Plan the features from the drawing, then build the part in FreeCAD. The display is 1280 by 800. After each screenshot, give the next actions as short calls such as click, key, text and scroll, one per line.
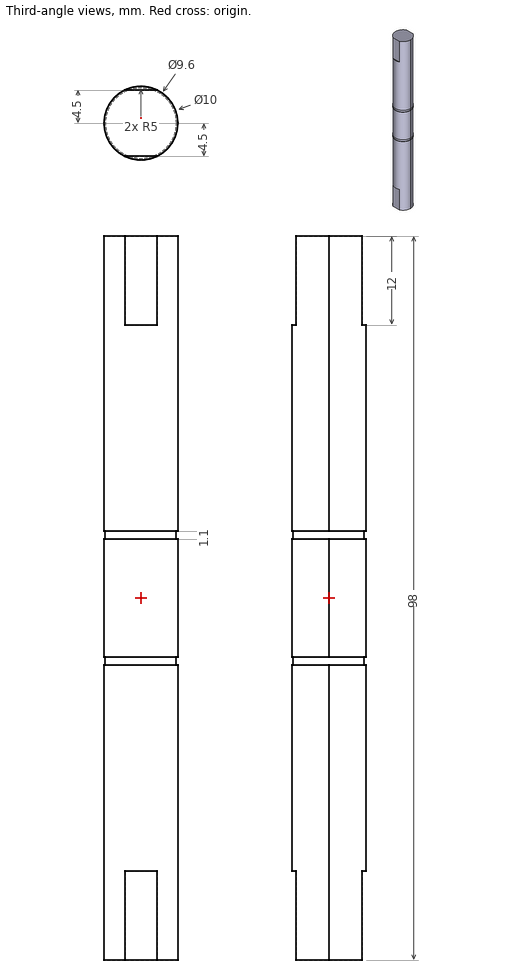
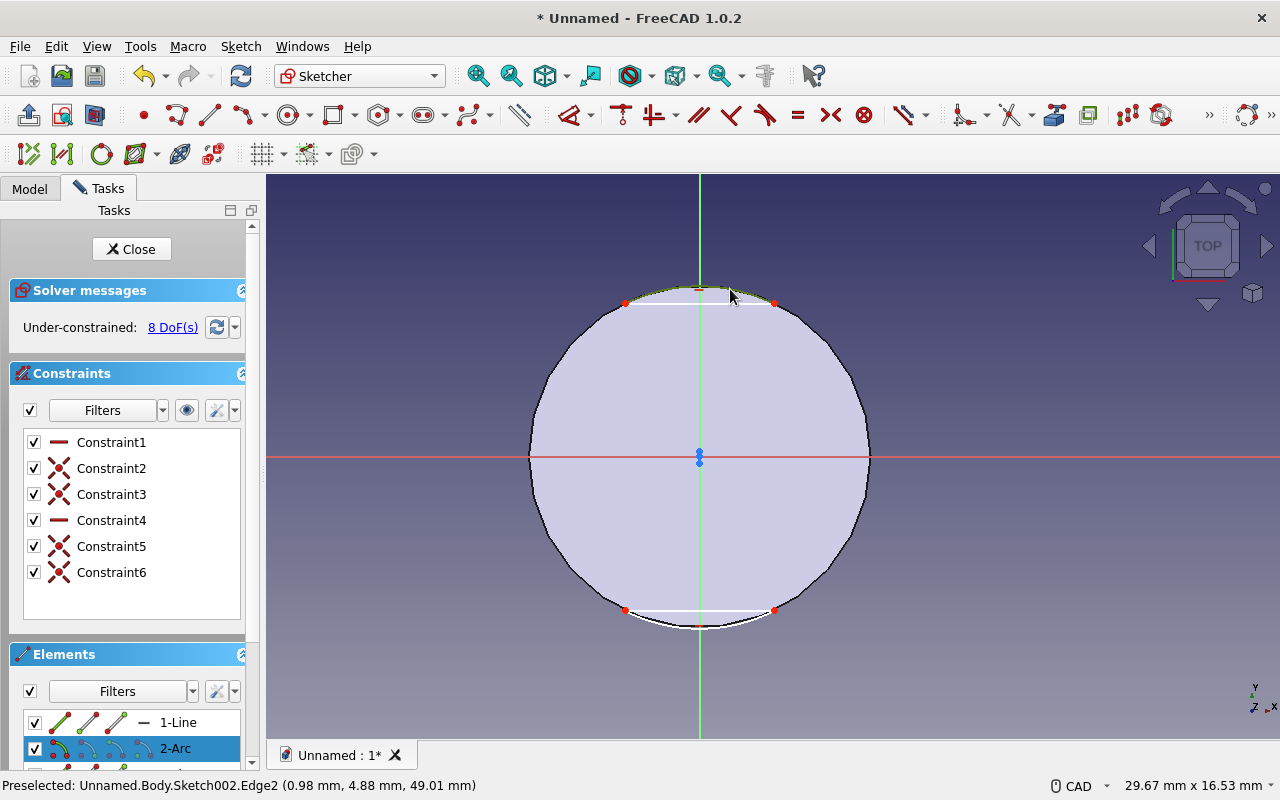
click(669, 626)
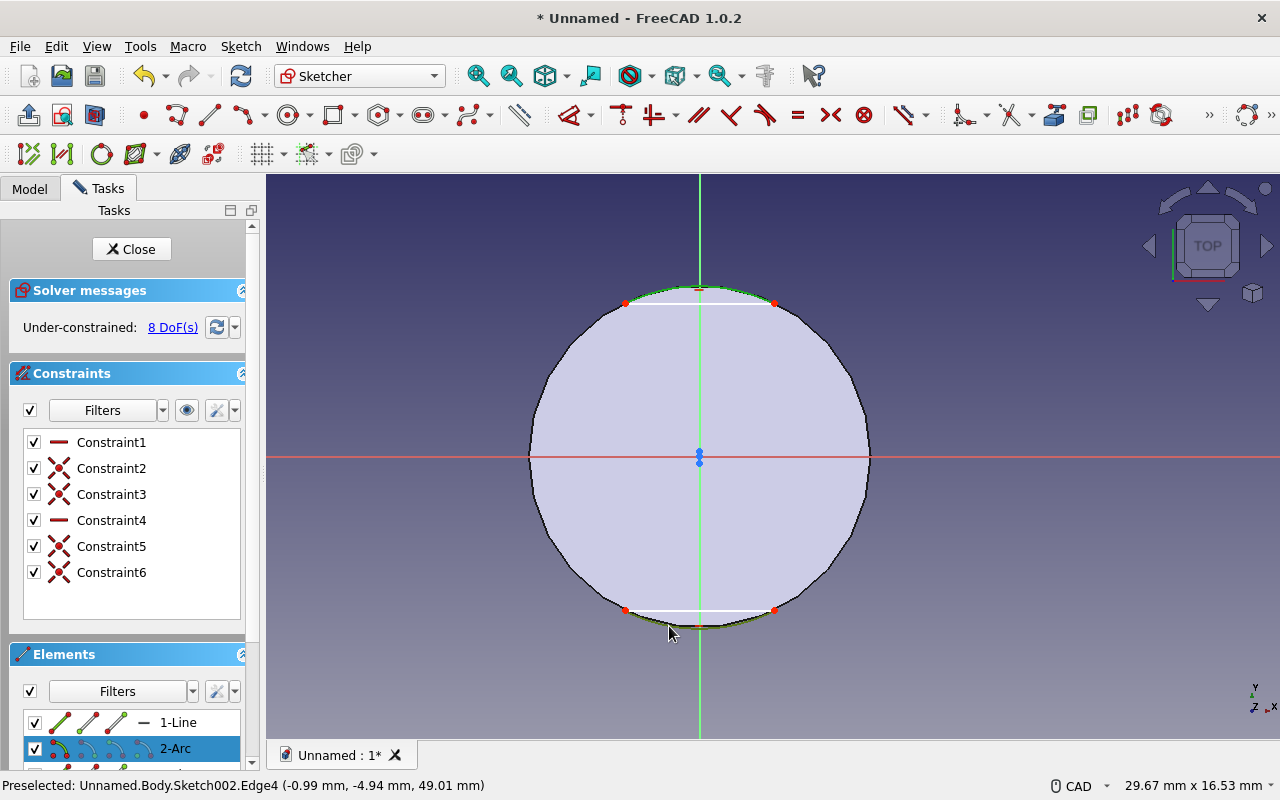
click(621, 116)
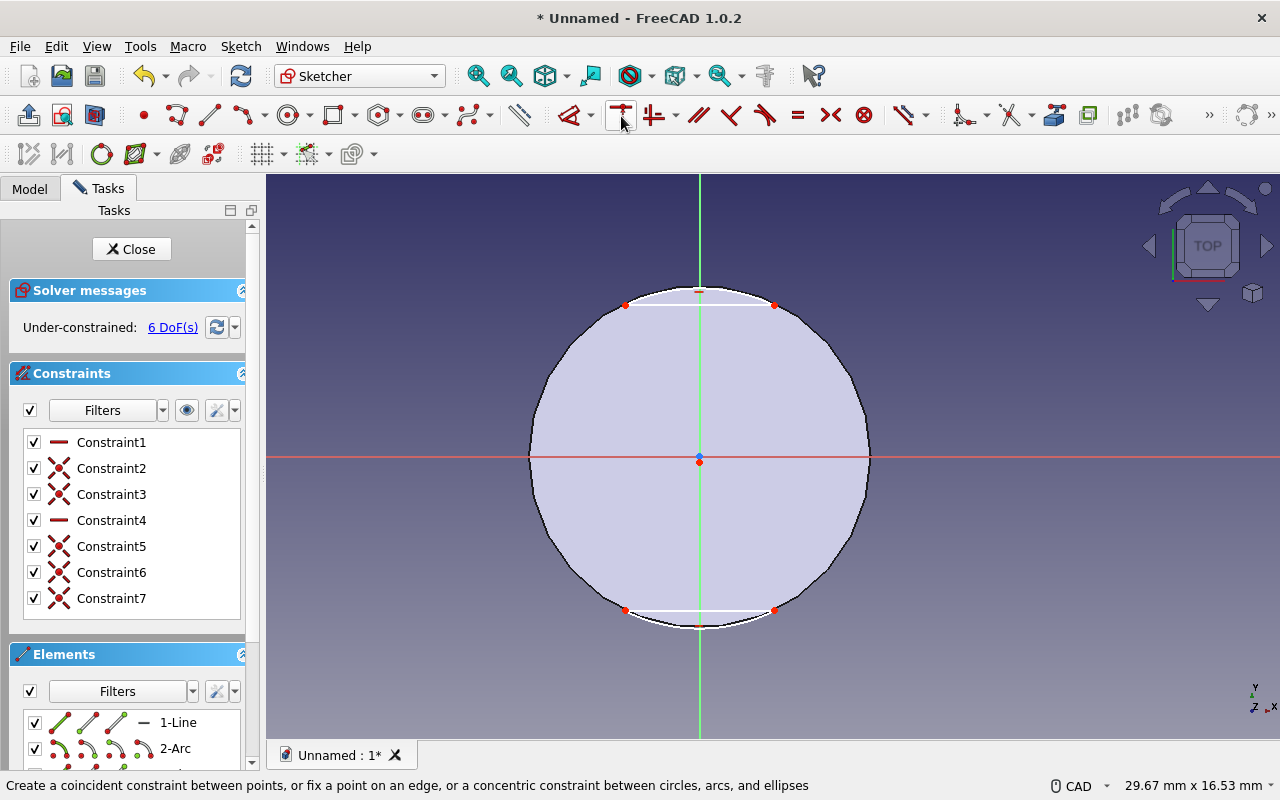
drag(690, 446, 710, 472)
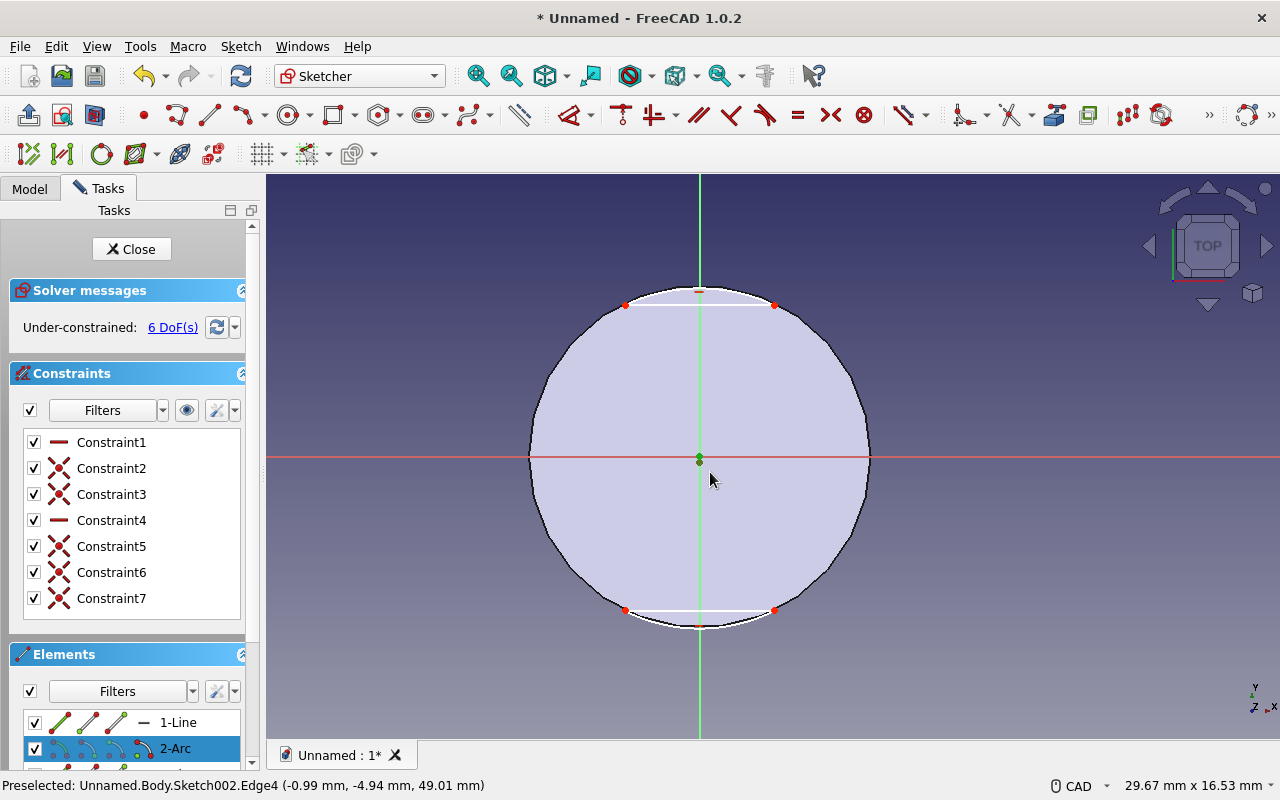
click(621, 116)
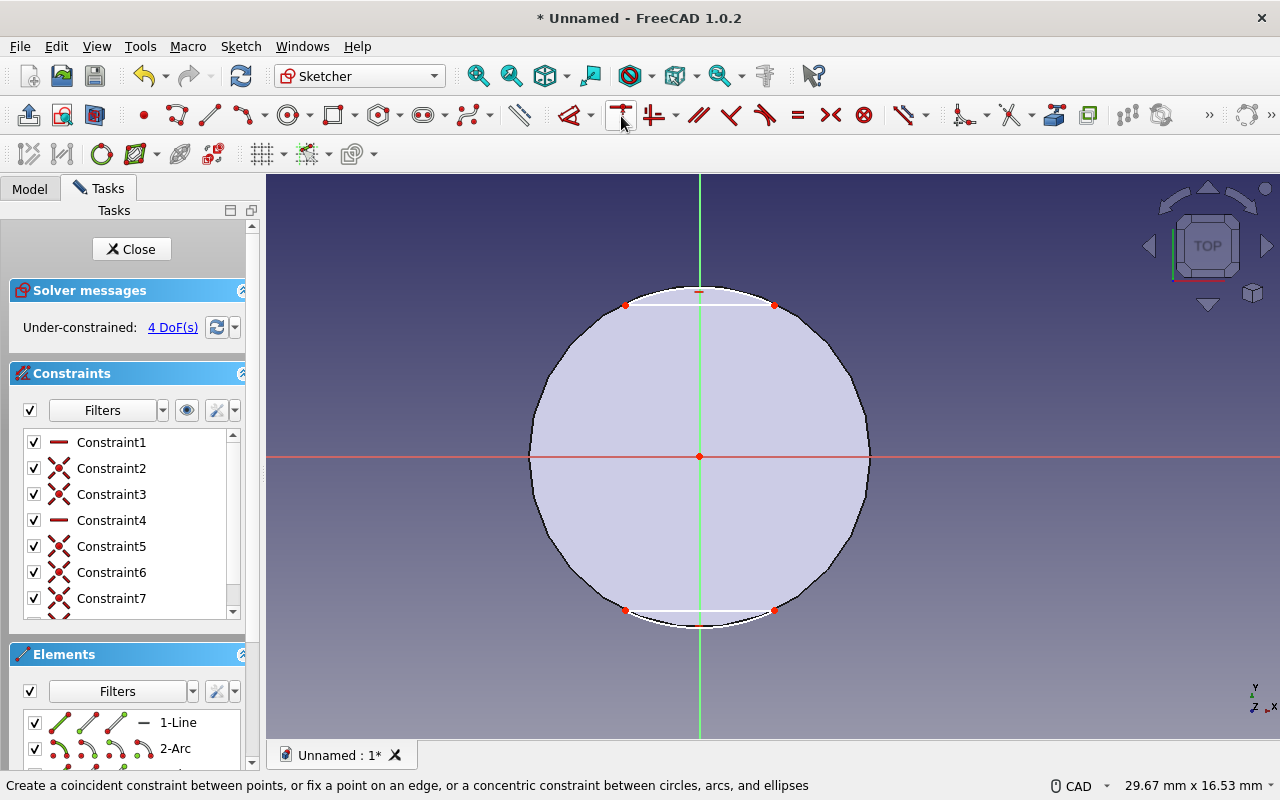
click(730, 291)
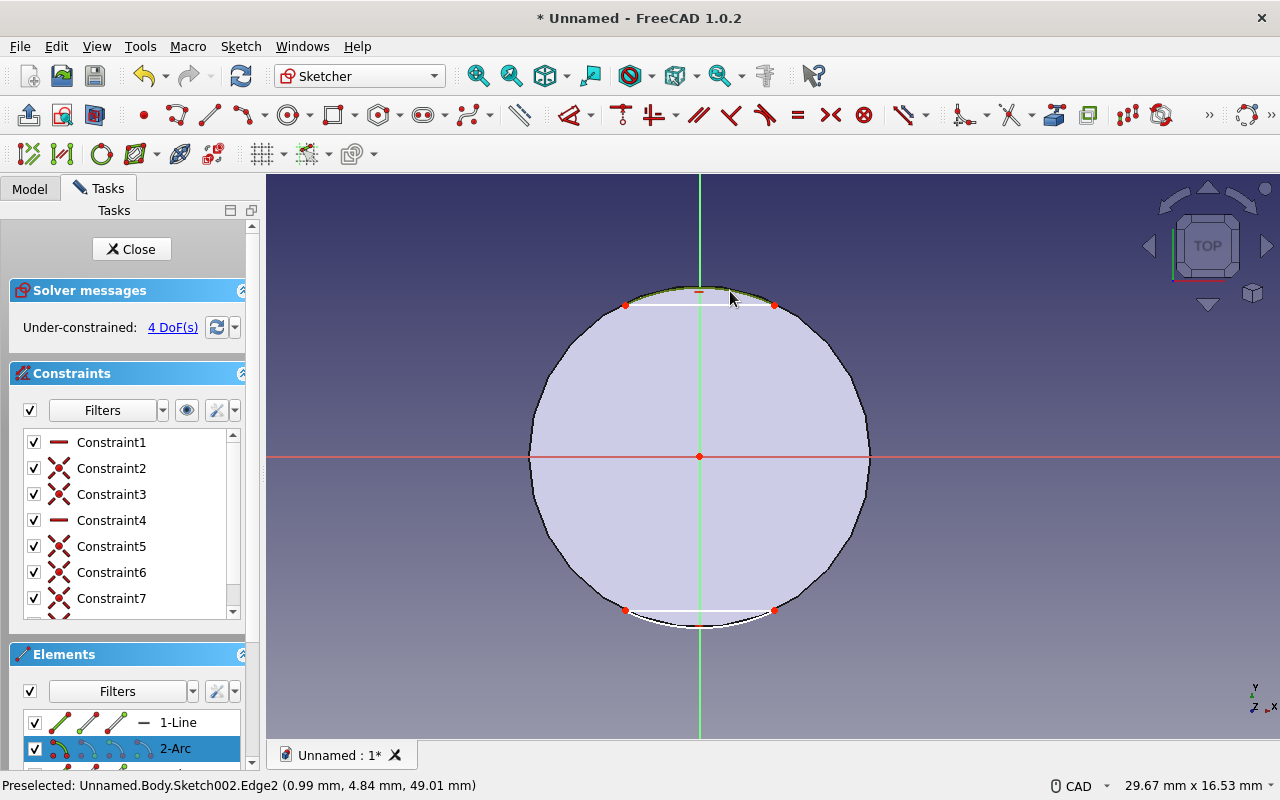
click(669, 625)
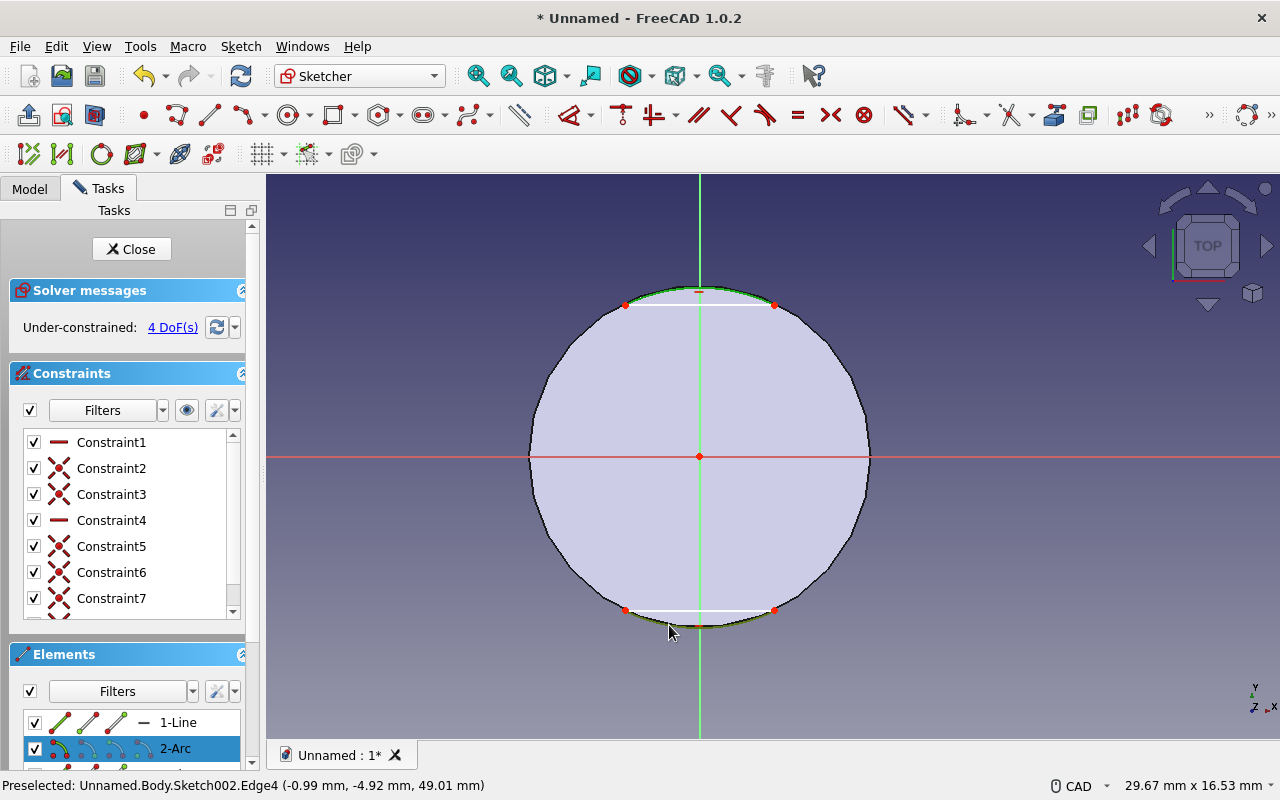
click(798, 116)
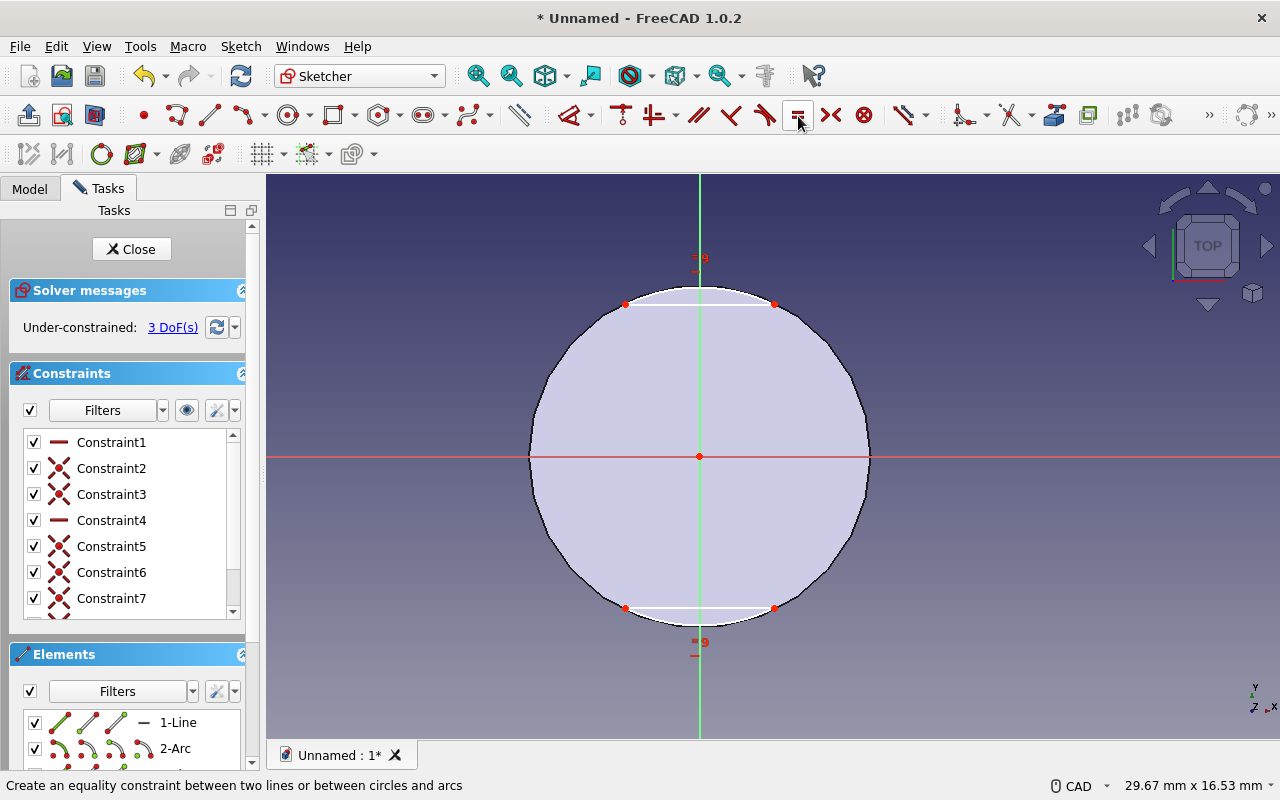
click(568, 116)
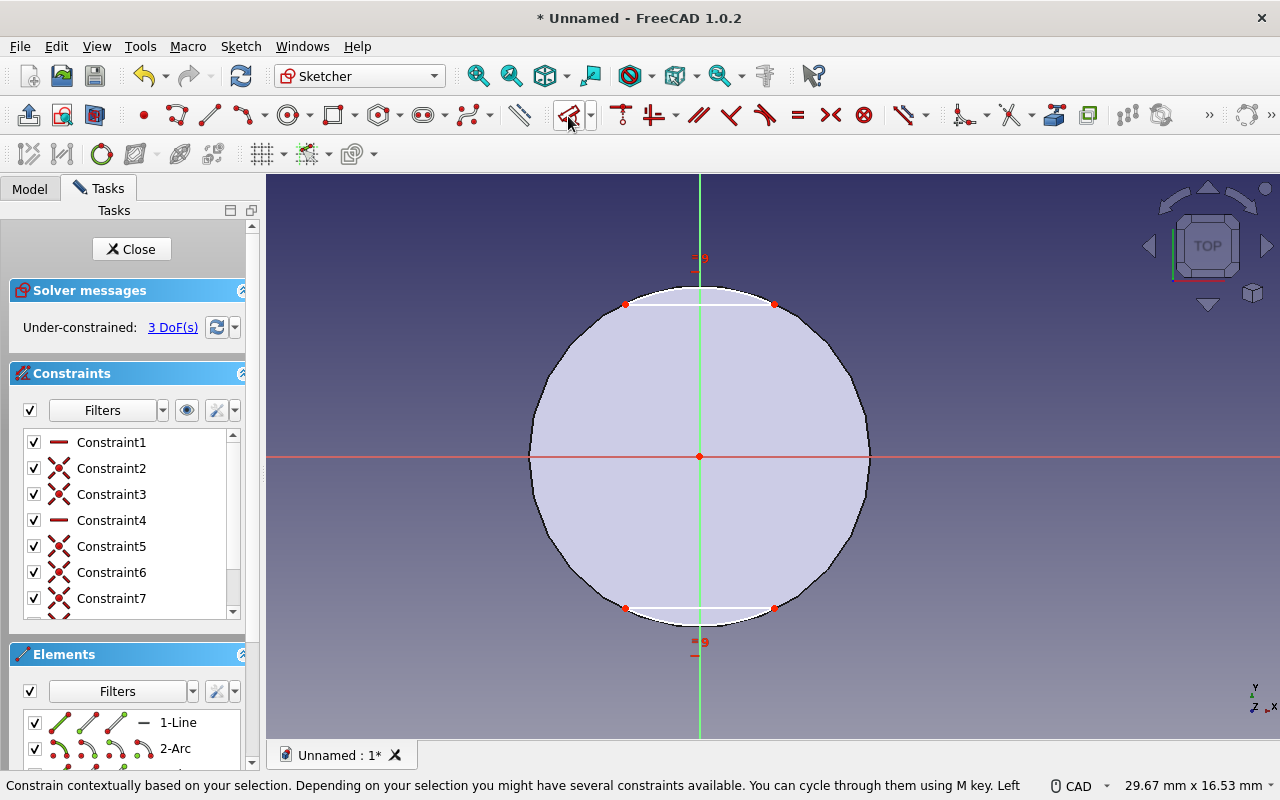
click(730, 290)
click(736, 259)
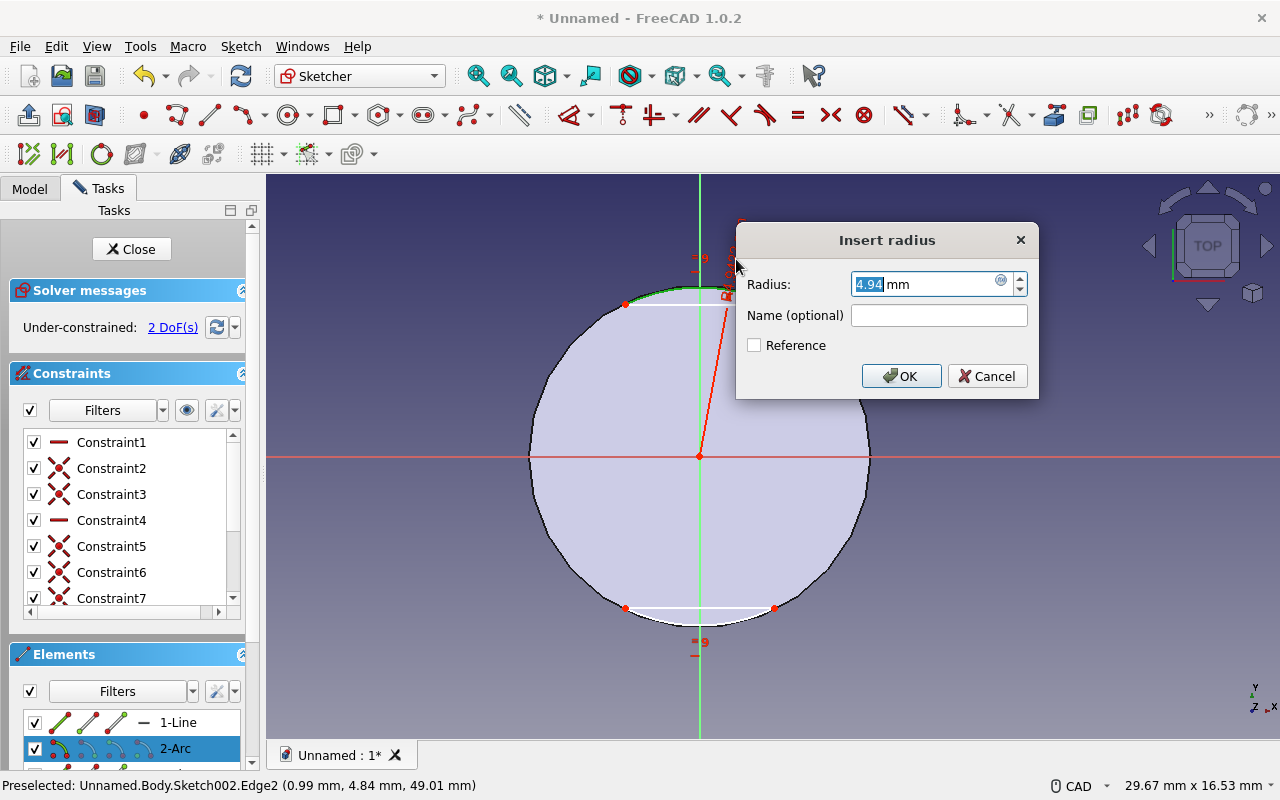
text(5)
key(Return)